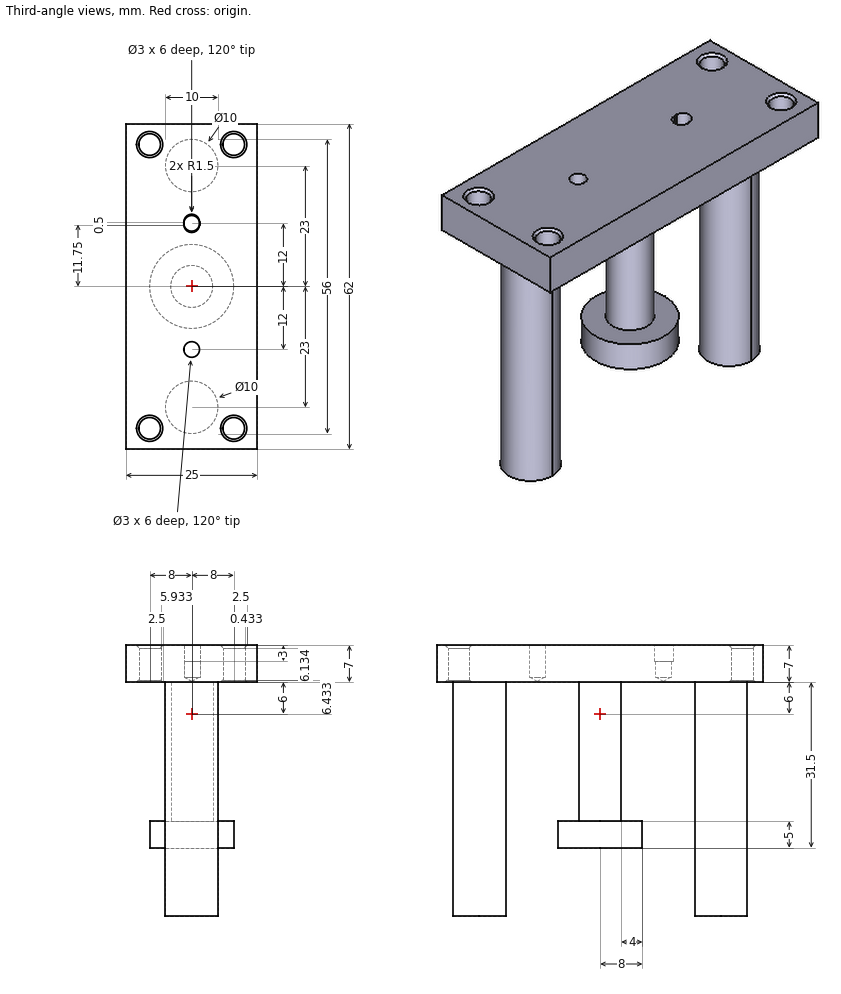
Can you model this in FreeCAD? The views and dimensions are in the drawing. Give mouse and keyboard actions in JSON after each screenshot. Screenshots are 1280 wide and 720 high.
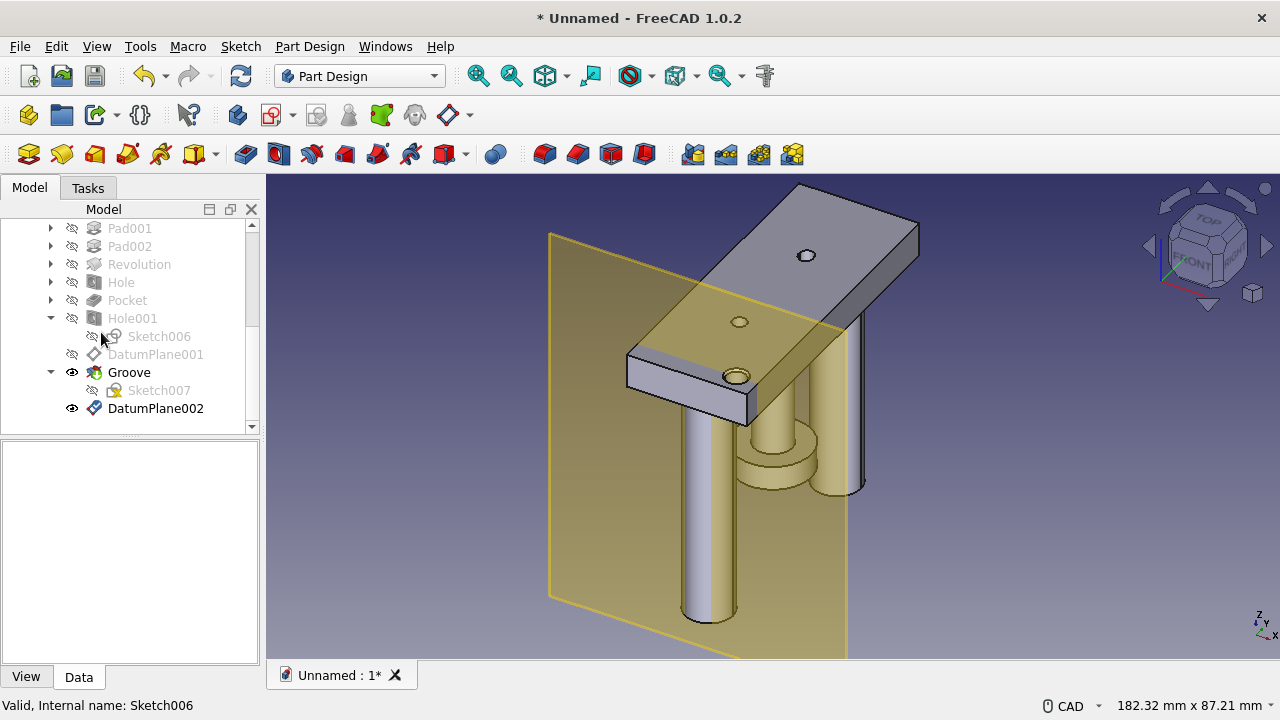
{"action": "left_click", "coordinate": [117, 408]}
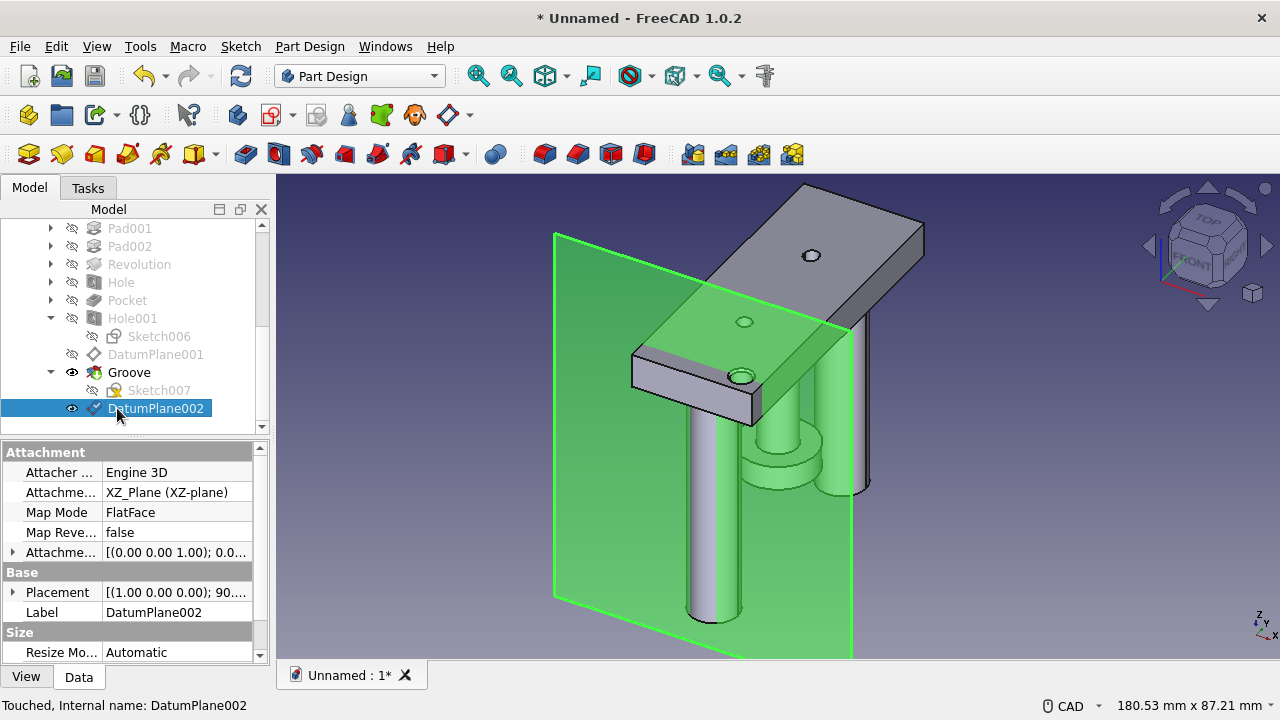
{"action": "left_click", "coordinate": [270, 116]}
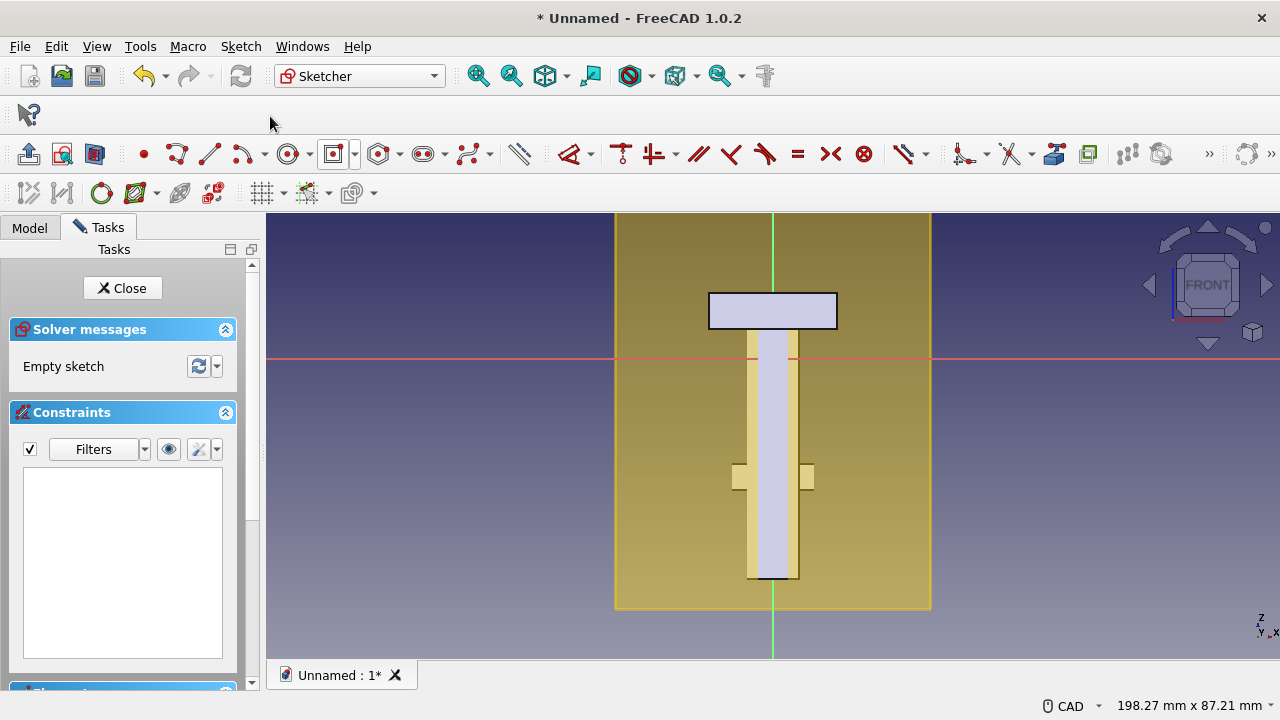
{"action": "left_click", "coordinate": [95, 154]}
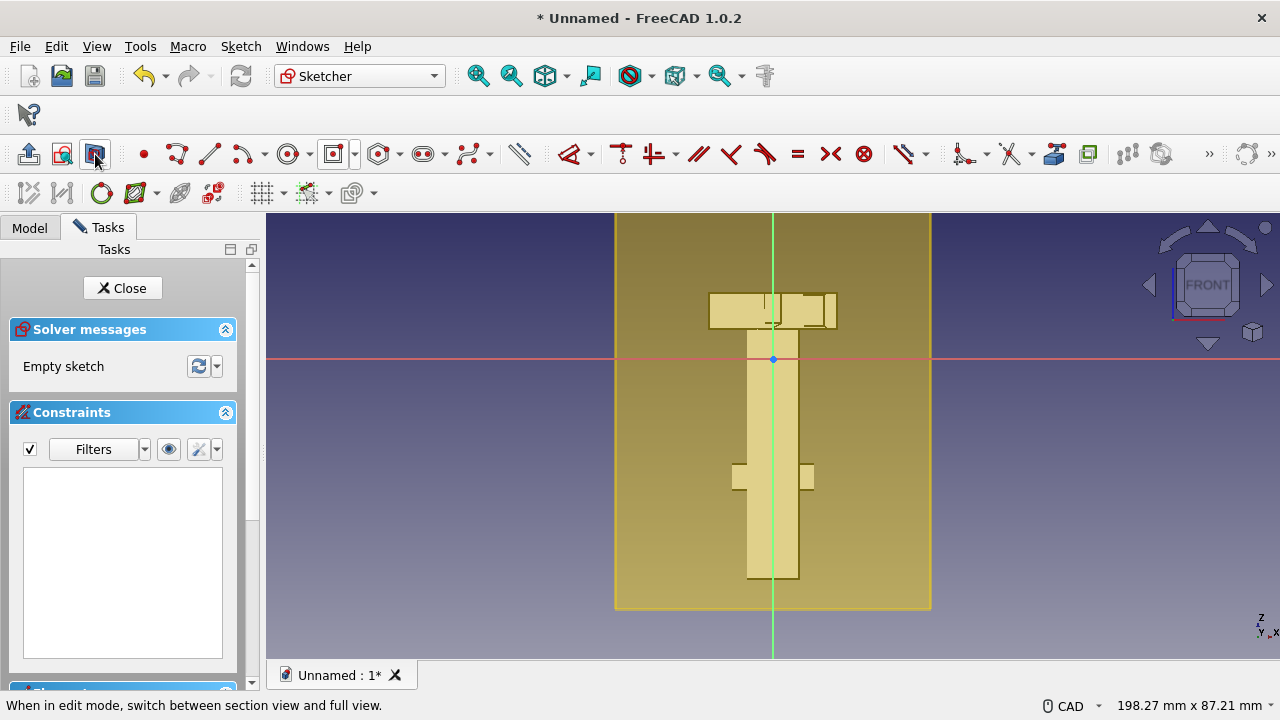
{"action": "scroll", "coordinate": [768, 290], "scroll_direction": "up", "scroll_amount": 7}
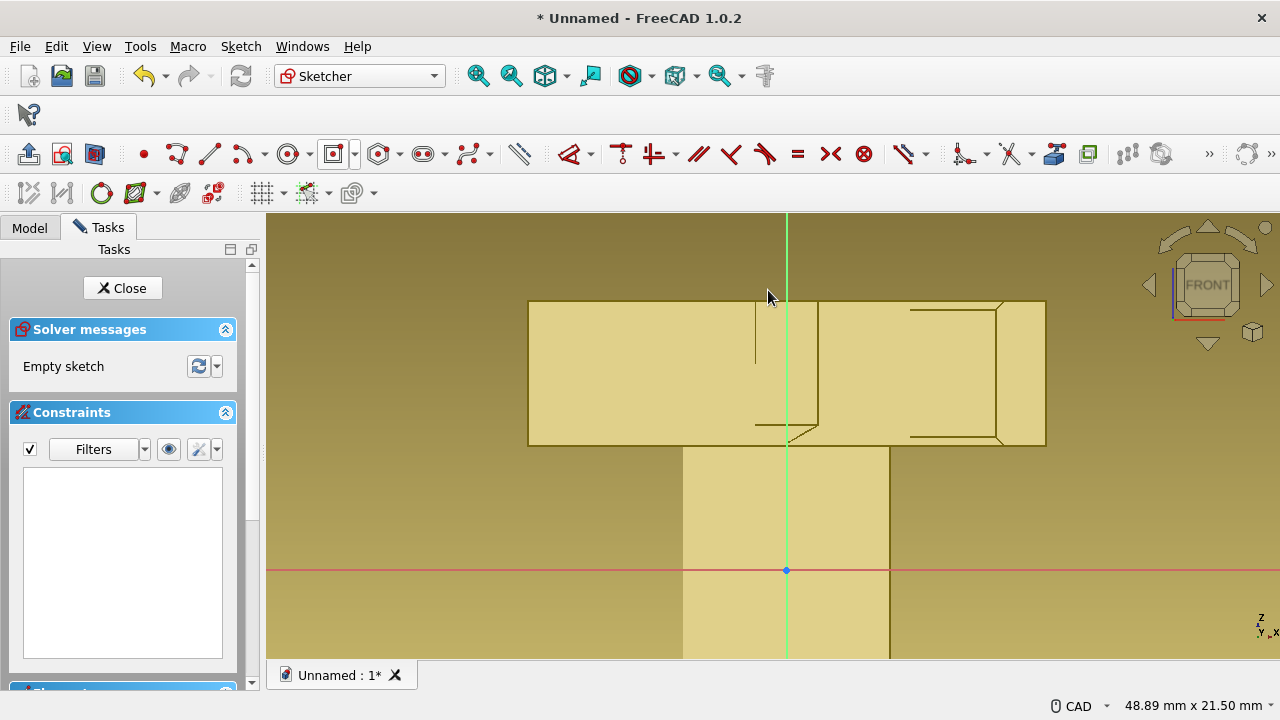
{"action": "left_click", "coordinate": [177, 154]}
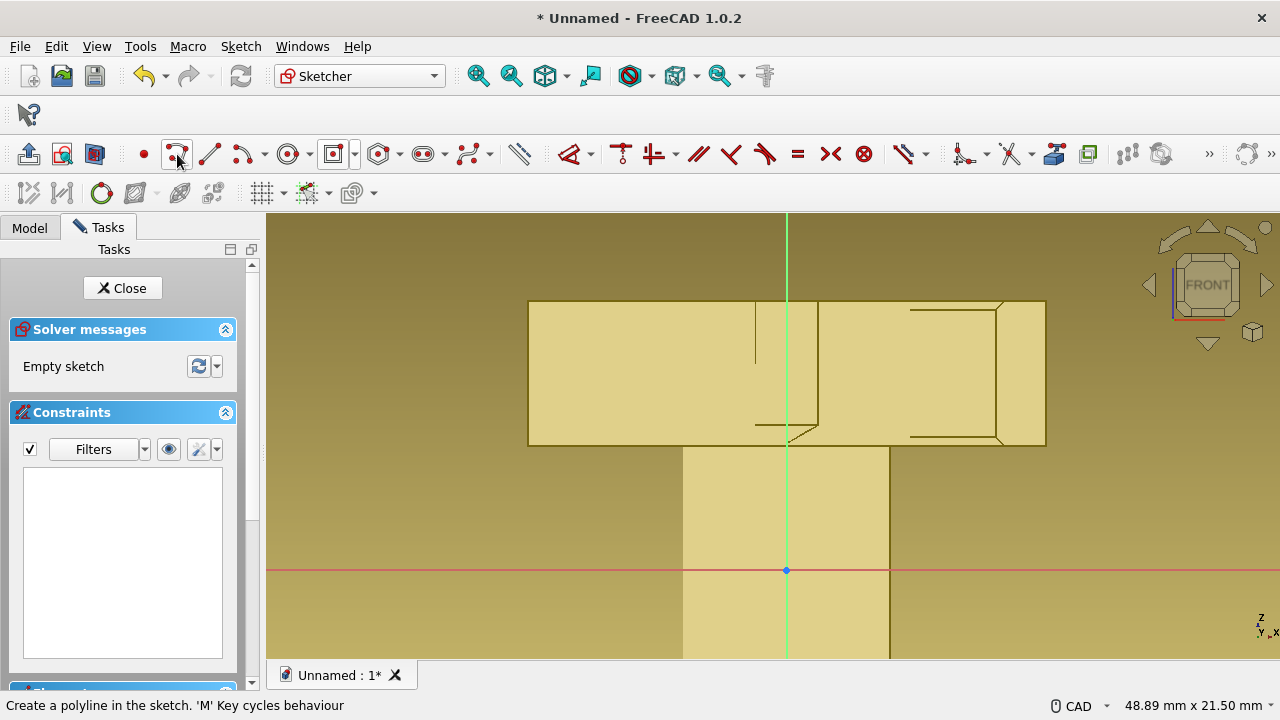
{"action": "left_click", "coordinate": [673, 446]}
{"action": "left_click", "coordinate": [621, 446]}
{"action": "left_click", "coordinate": [621, 301]}
{"action": "left_click", "coordinate": [673, 301]}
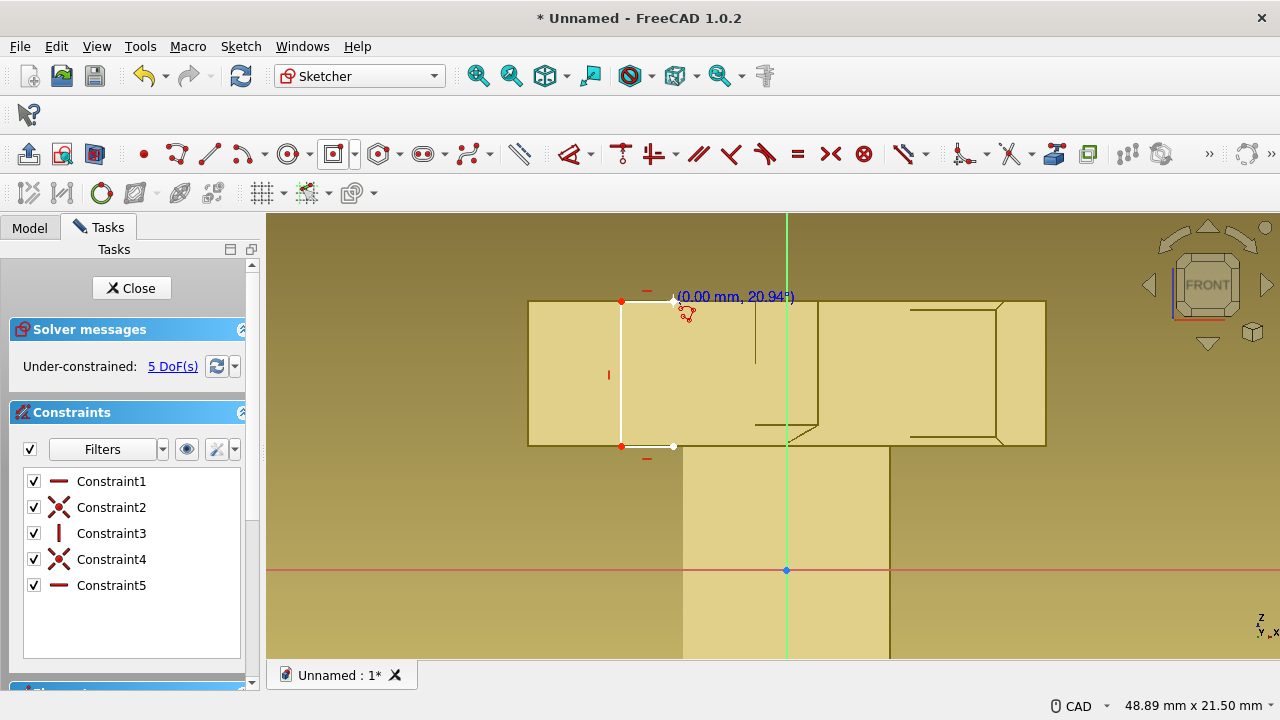
{"action": "scroll", "coordinate": [664, 310], "scroll_direction": "up", "scroll_amount": 3}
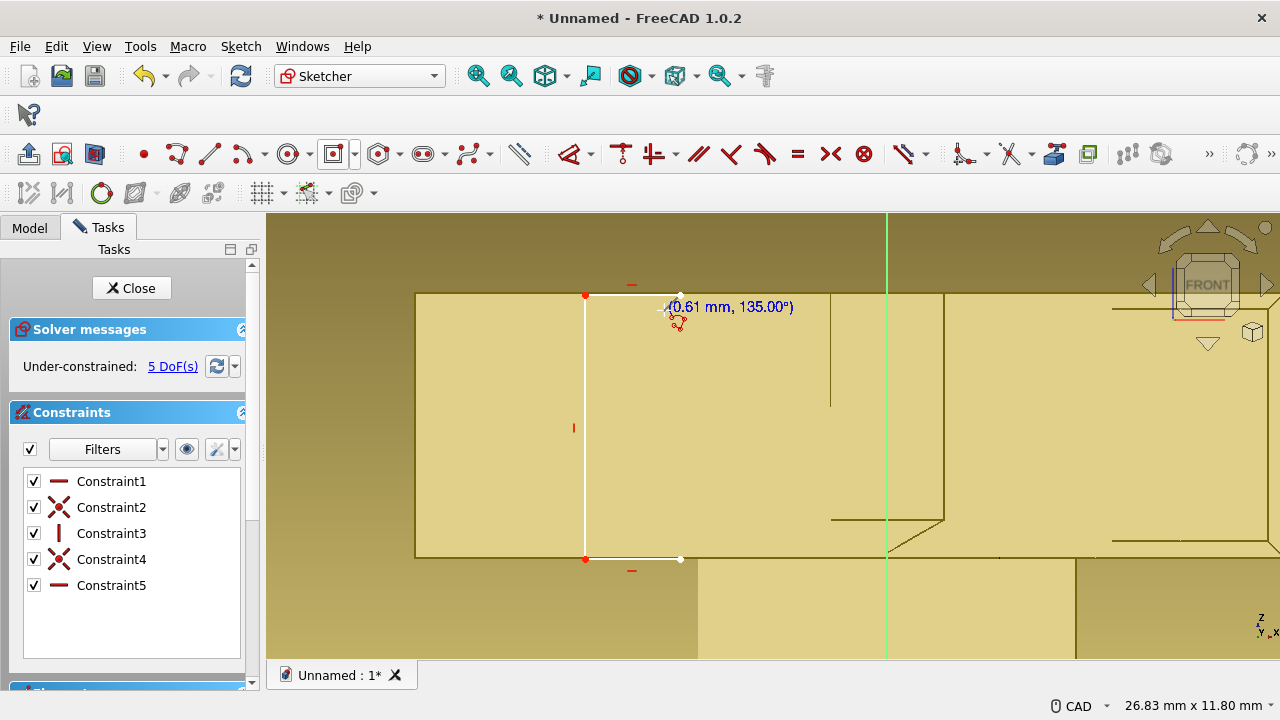
{"action": "left_click", "coordinate": [663, 309]}
{"action": "left_click", "coordinate": [663, 541]}
{"action": "left_click", "coordinate": [680, 559]}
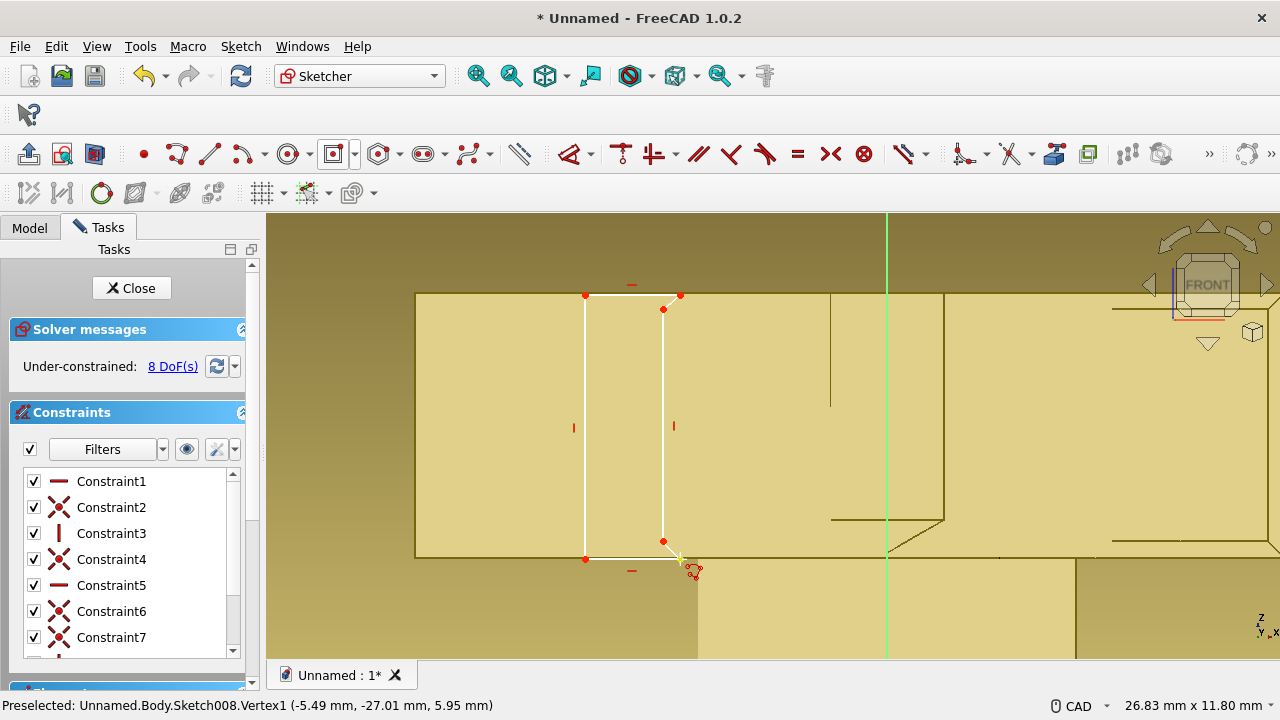
{"action": "left_click", "coordinate": [210, 154]}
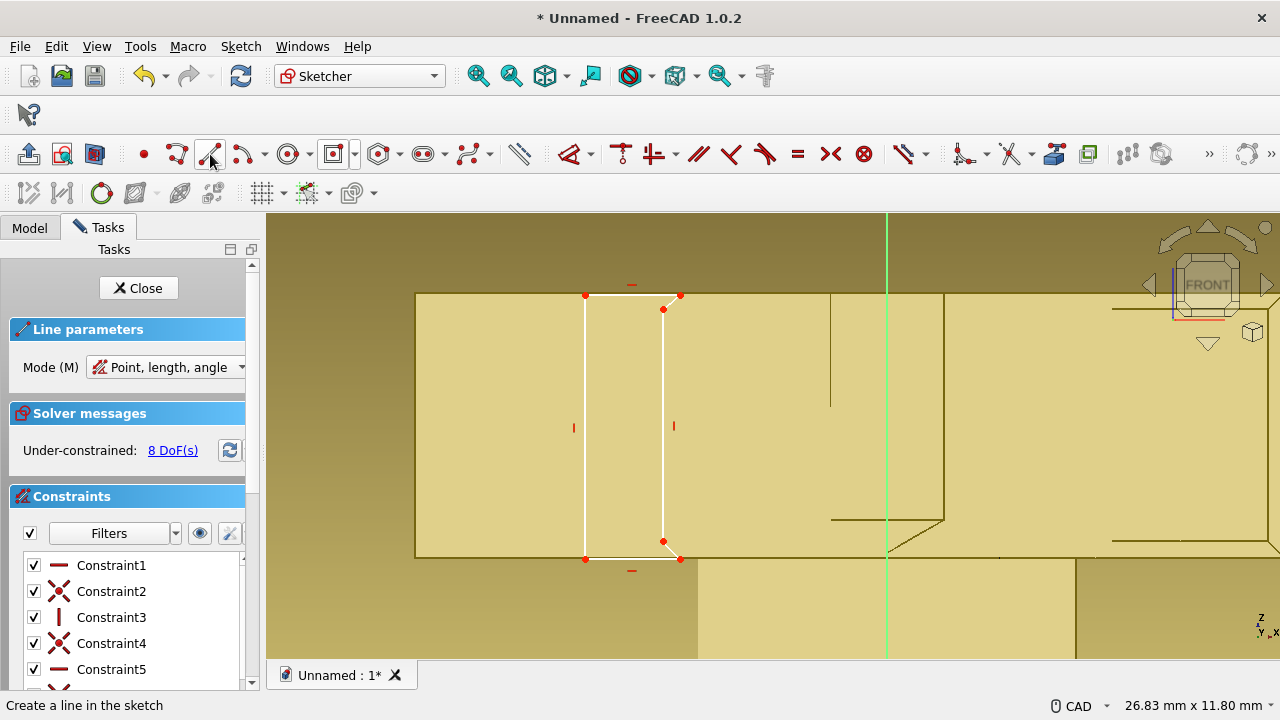
{"action": "left_click", "coordinate": [585, 584]}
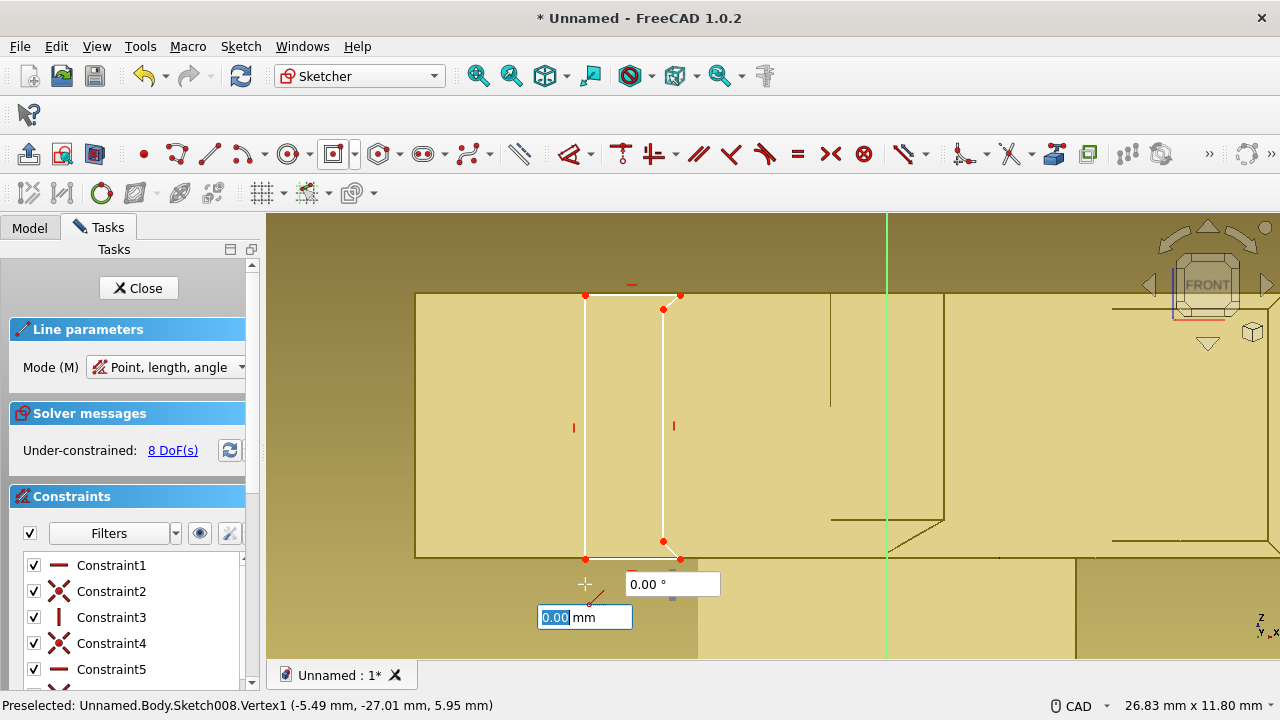
{"action": "scroll", "coordinate": [666, 311], "scroll_direction": "down", "scroll_amount": 3}